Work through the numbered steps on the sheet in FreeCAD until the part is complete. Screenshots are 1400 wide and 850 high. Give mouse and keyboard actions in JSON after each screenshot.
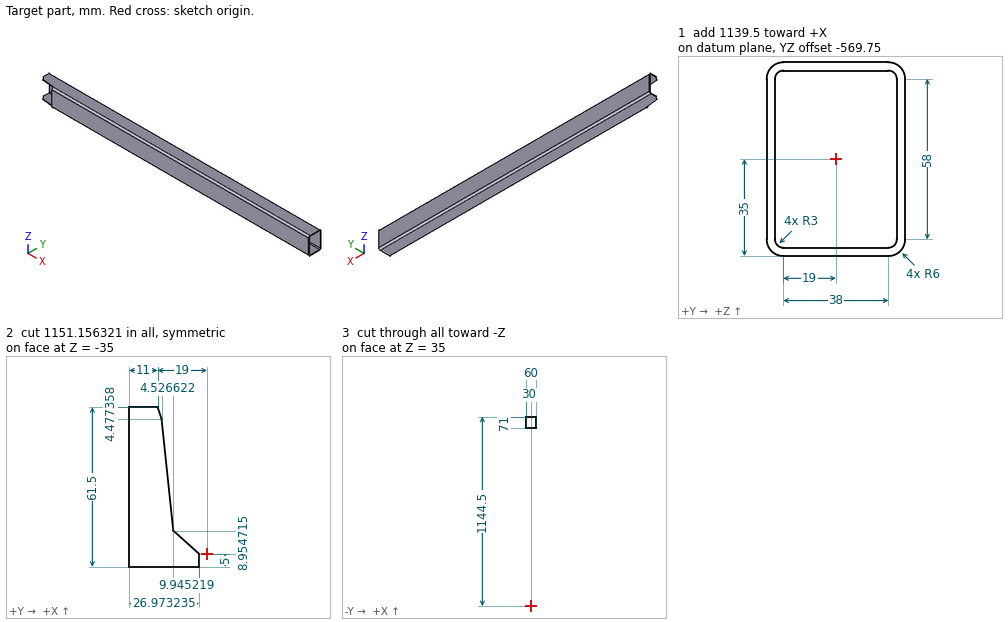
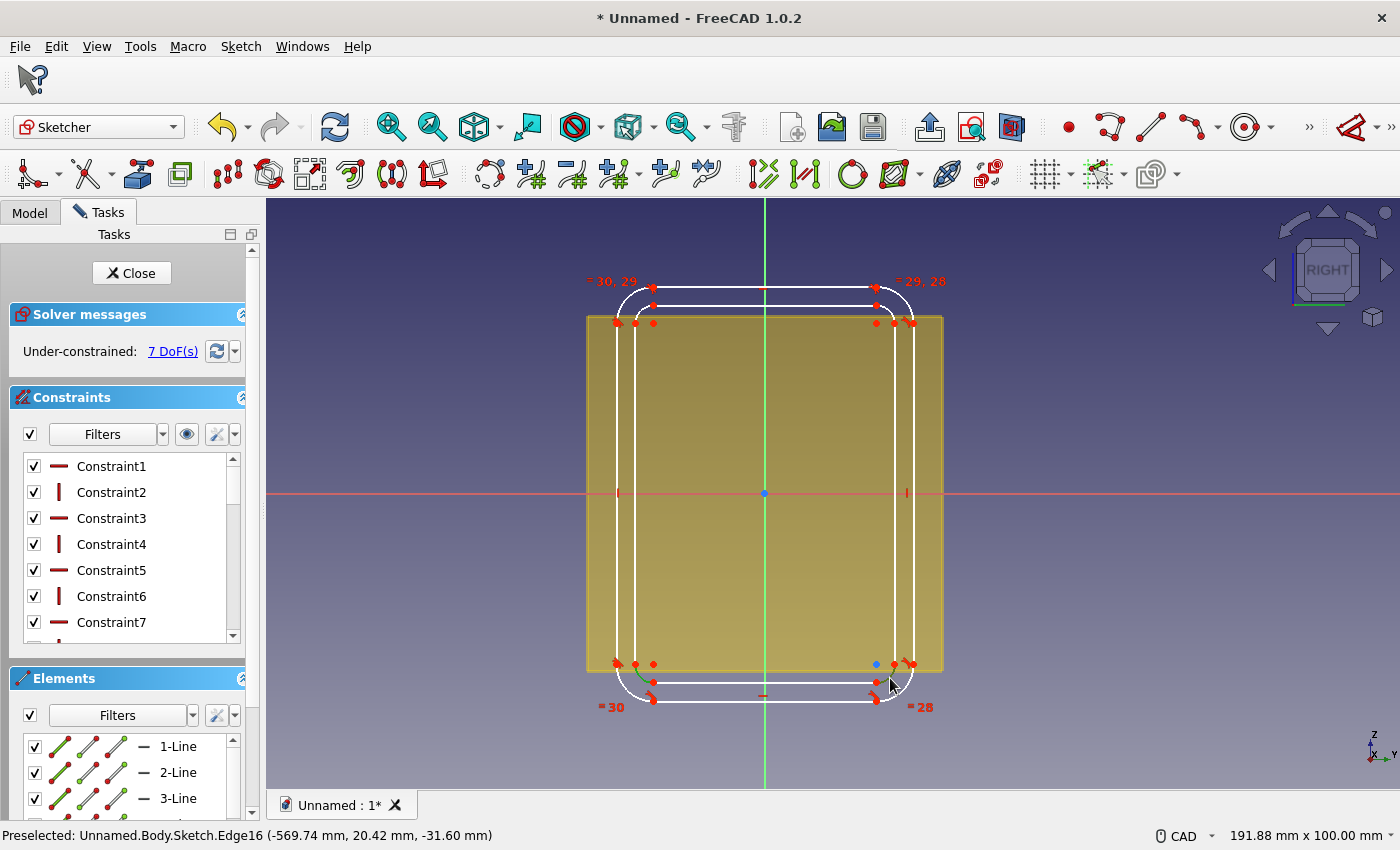
{"action": "key", "text": "e"}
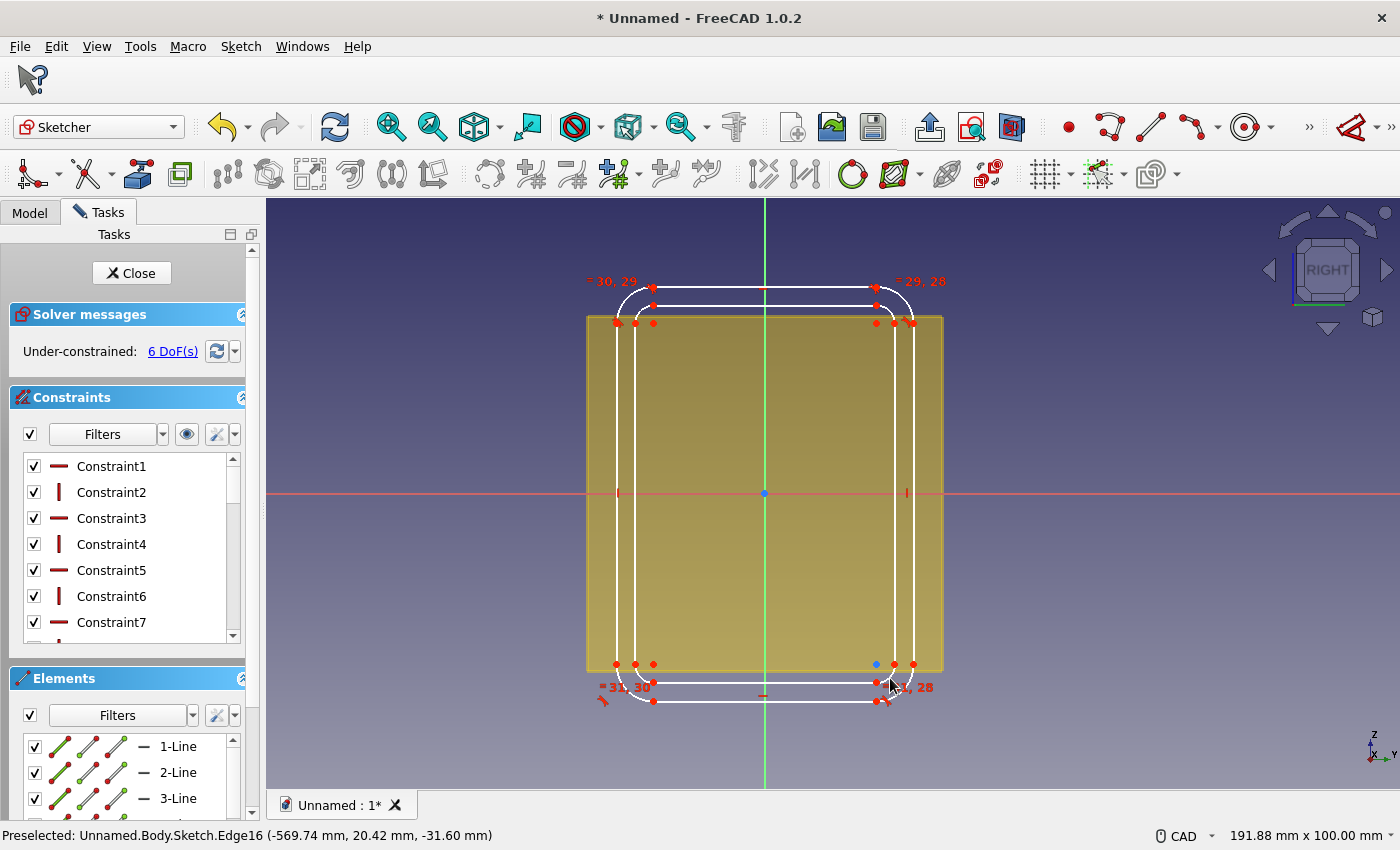
{"action": "left_click", "coordinate": [912, 676]}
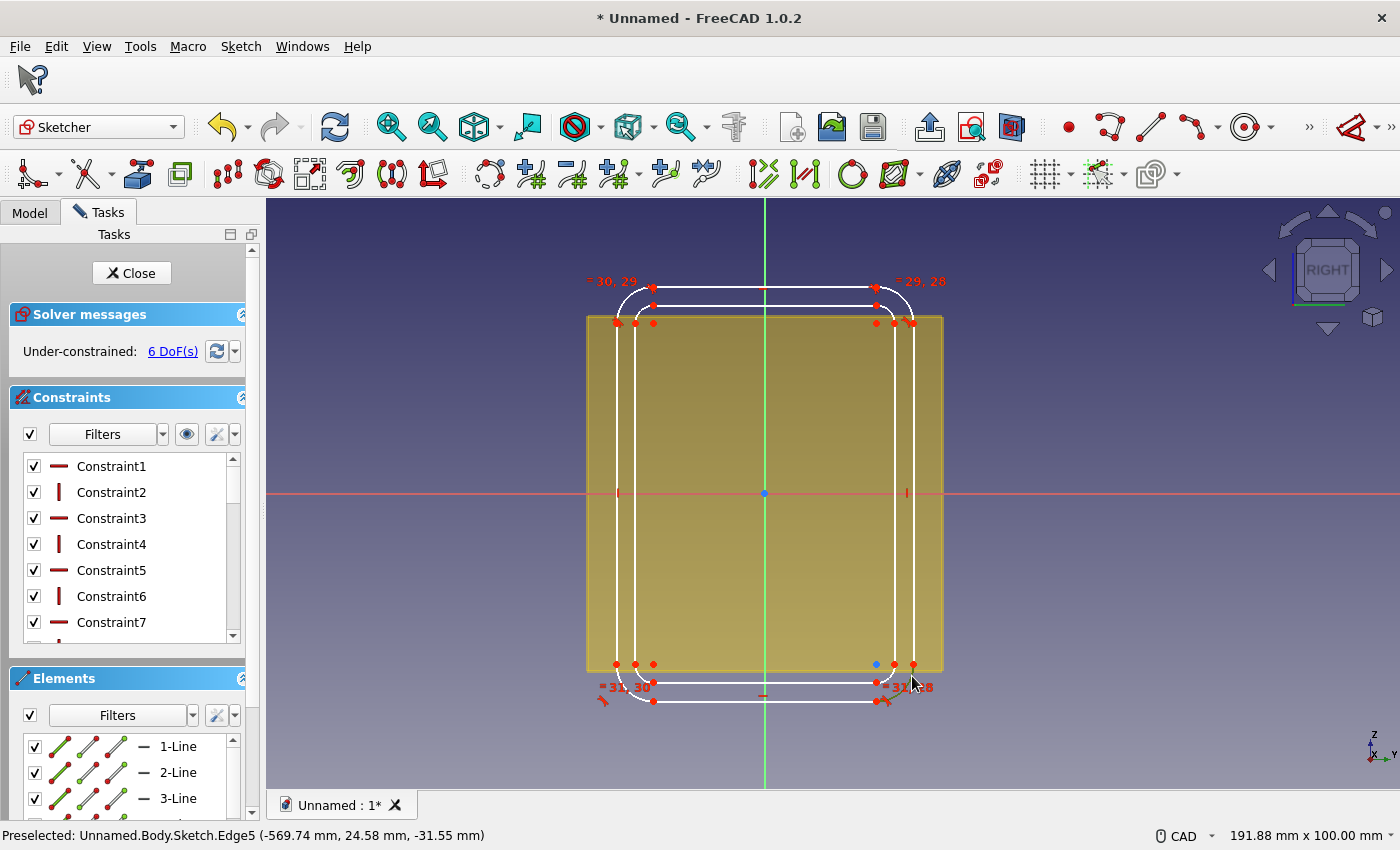
{"action": "key", "text": "k r"}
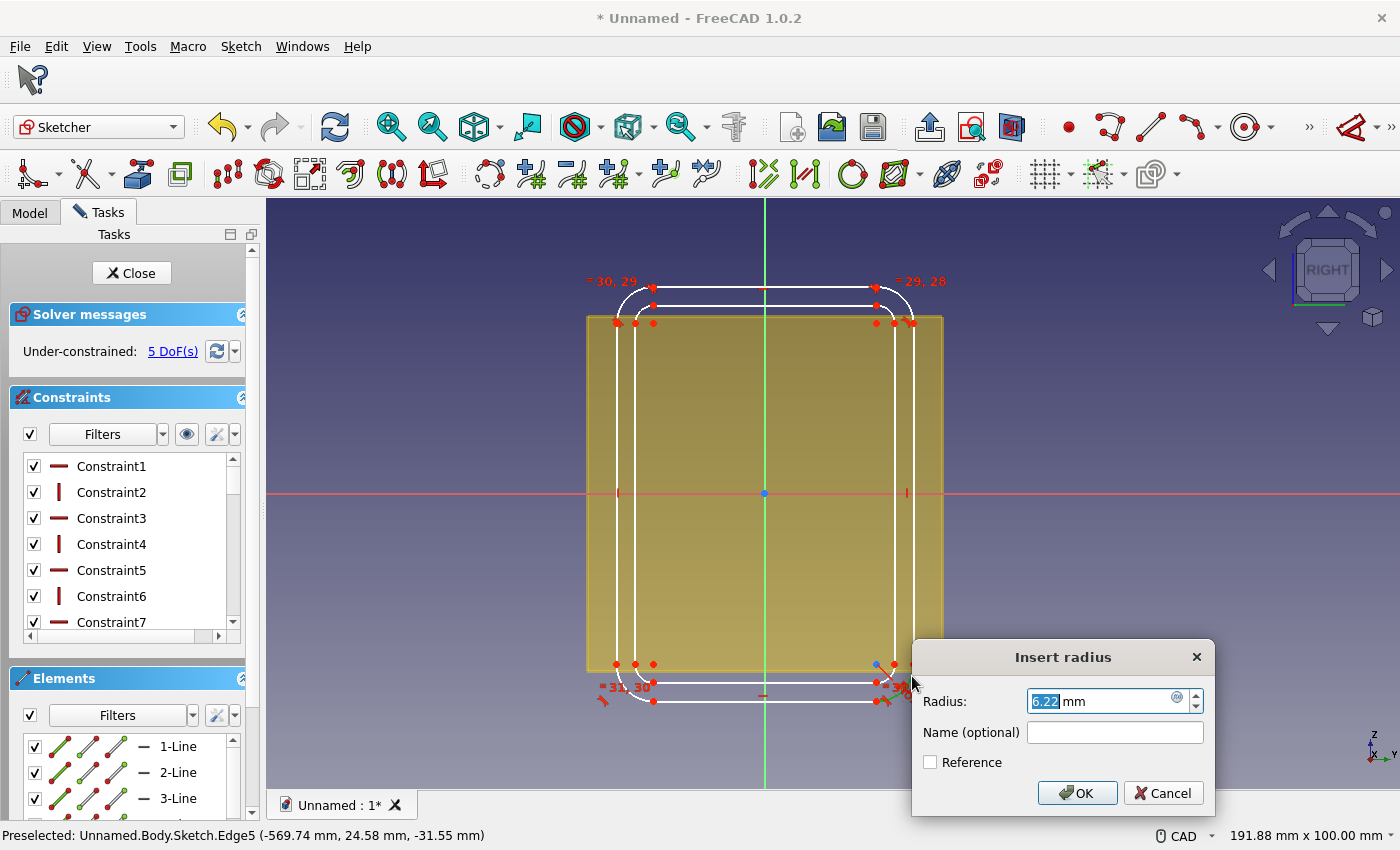
{"action": "type", "text": "6"}
{"action": "key", "text": "Return"}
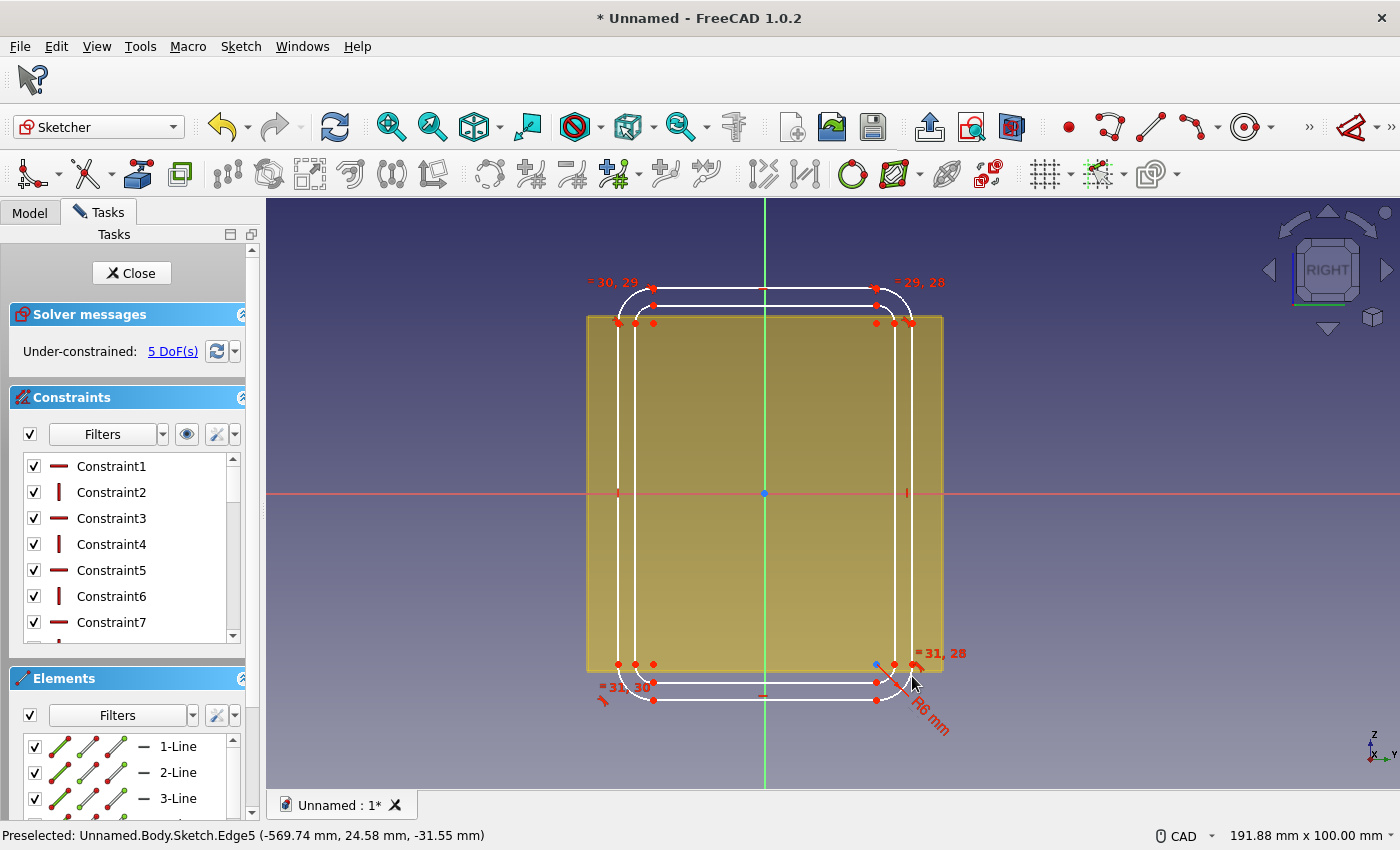
{"action": "scroll", "coordinate": [641, 678], "scroll_direction": "up", "scroll_amount": 5}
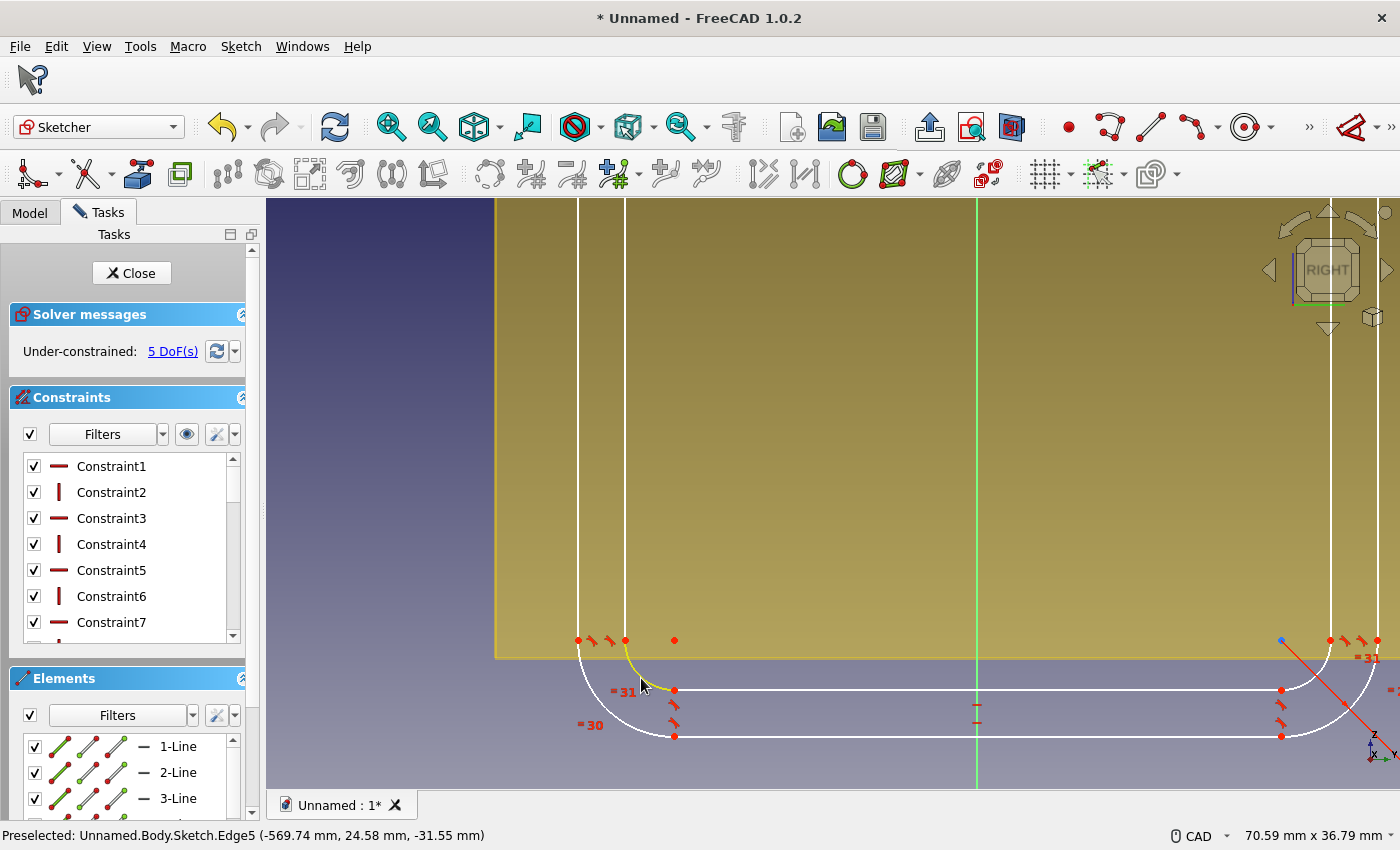
{"action": "left_click", "coordinate": [640, 676]}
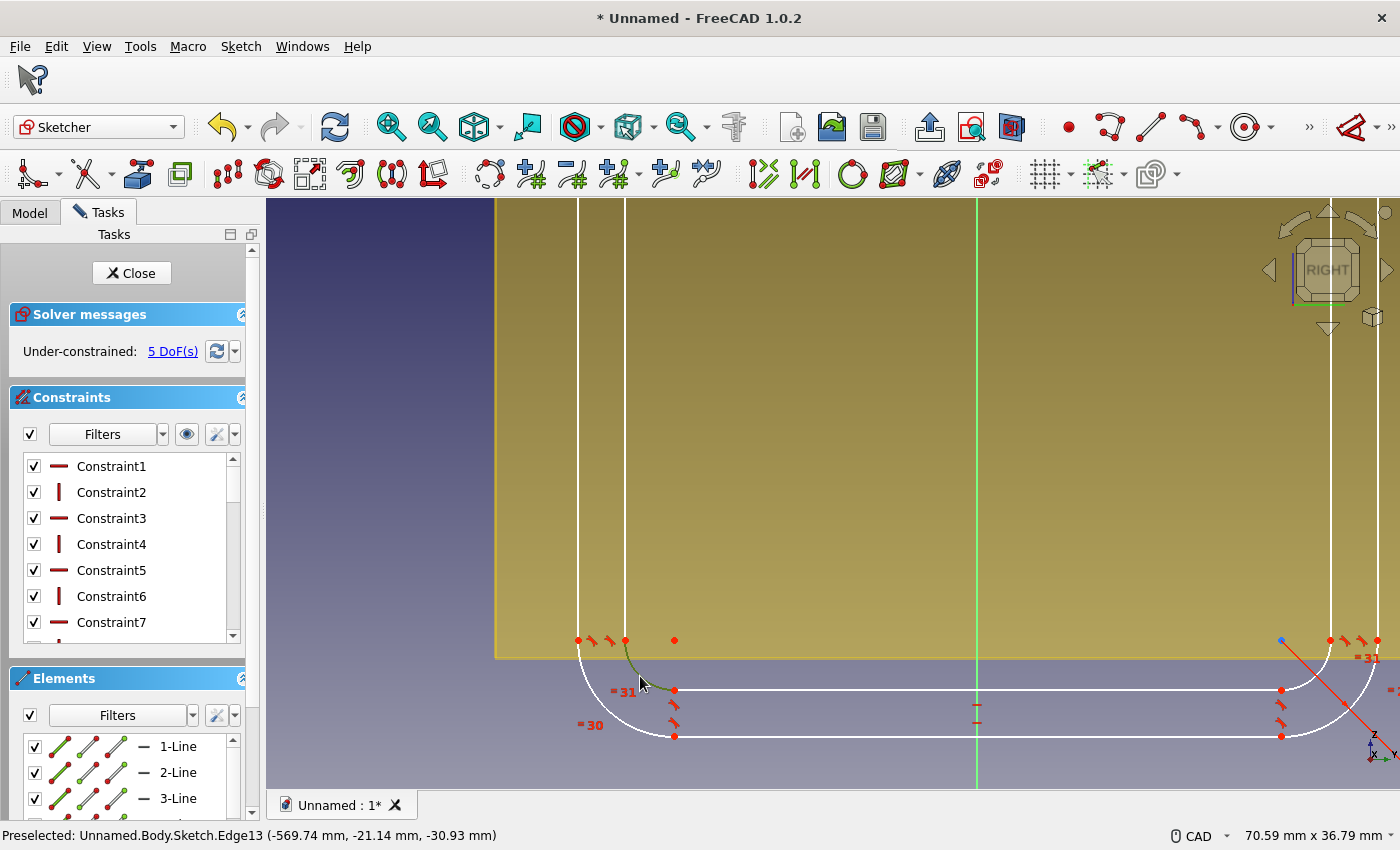
{"action": "key", "text": "k r"}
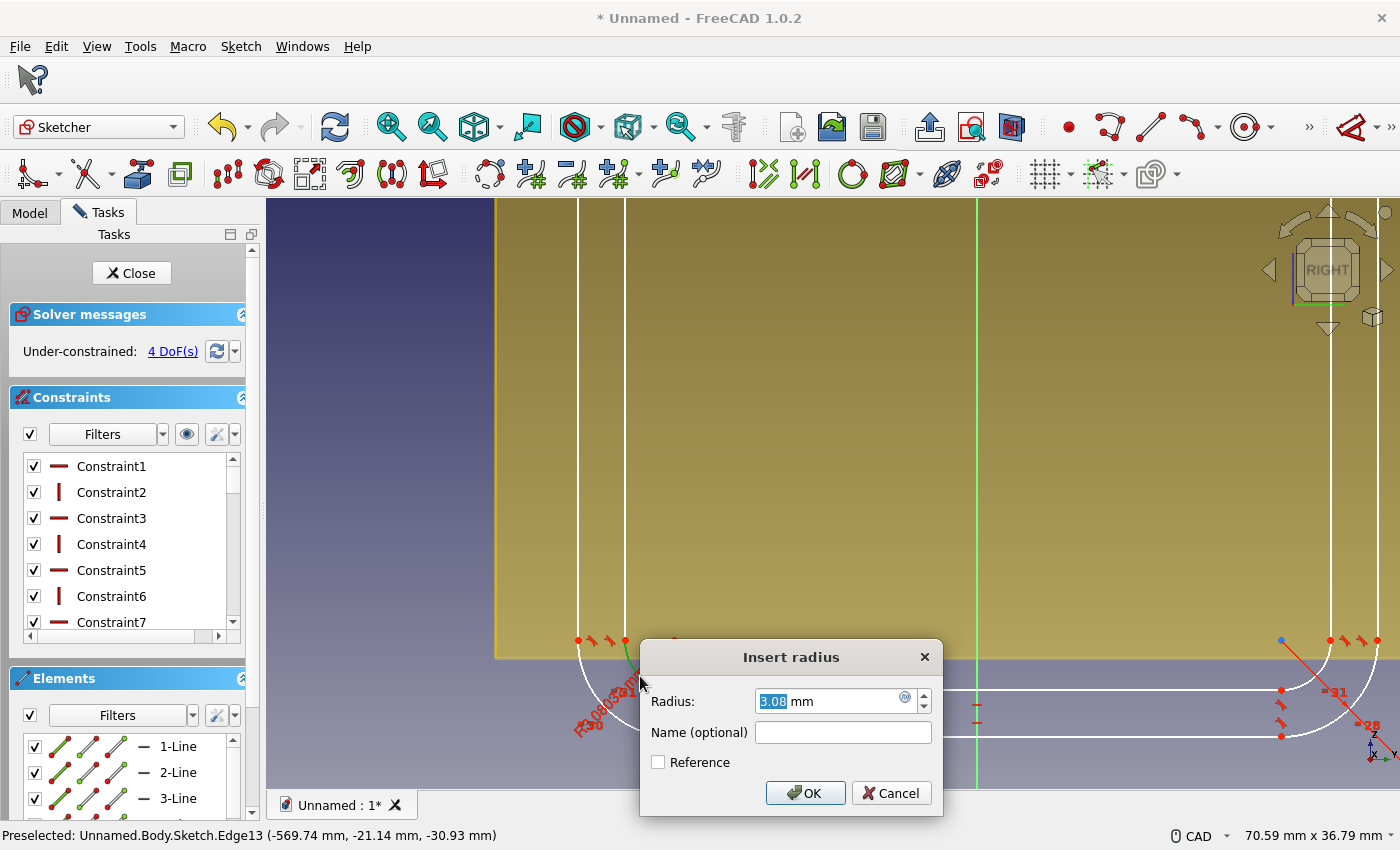
{"action": "type", "text": "3"}
{"action": "key", "text": "Return"}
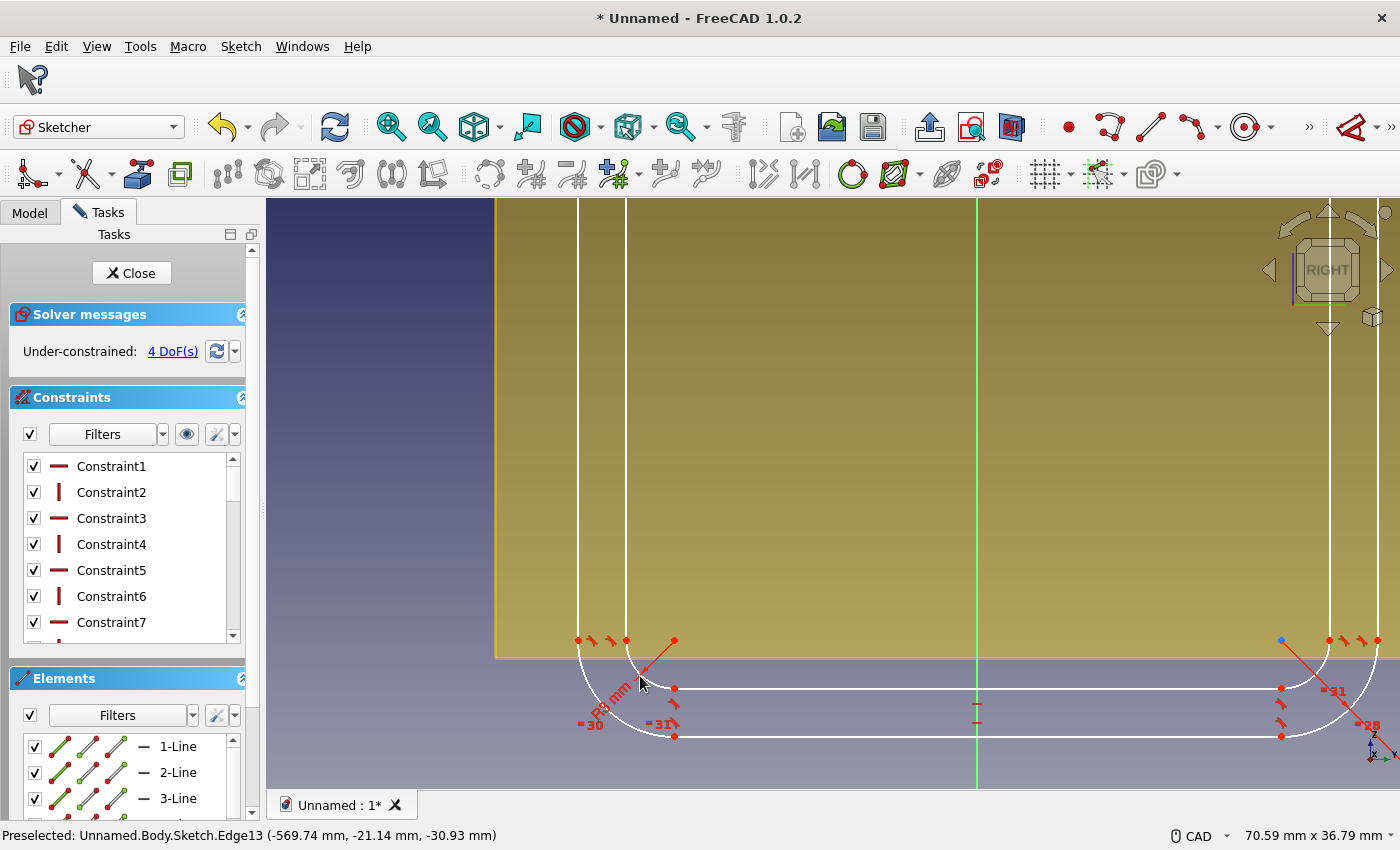
{"action": "left_click", "coordinate": [857, 737]}